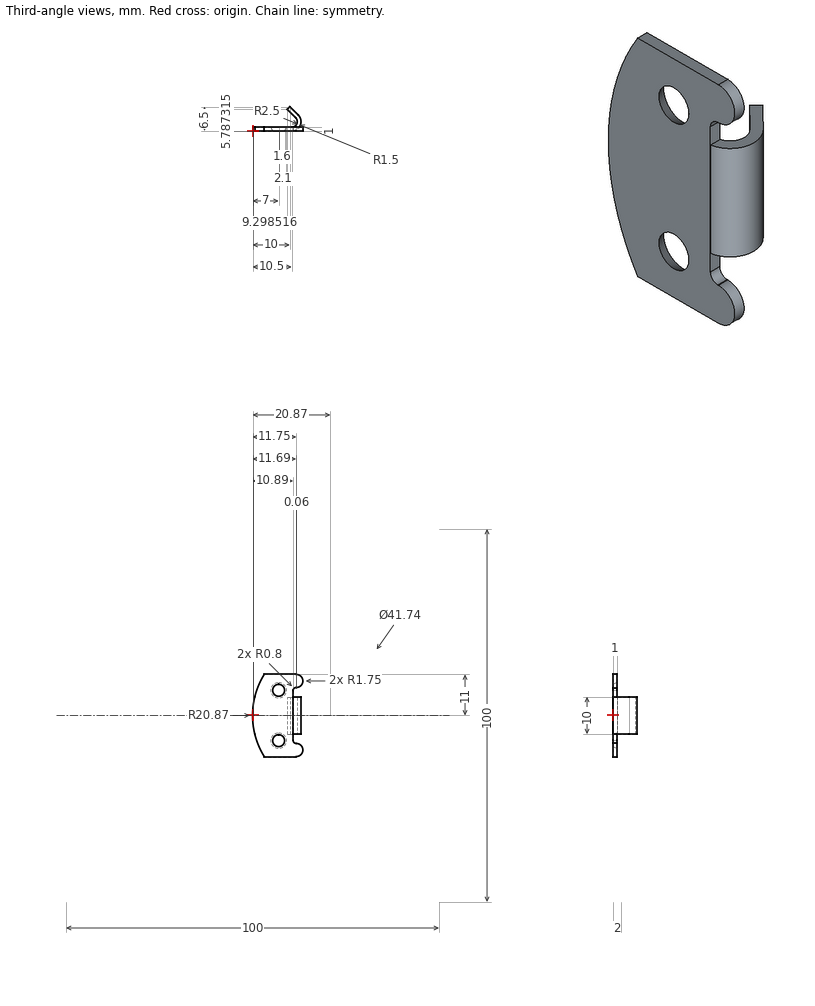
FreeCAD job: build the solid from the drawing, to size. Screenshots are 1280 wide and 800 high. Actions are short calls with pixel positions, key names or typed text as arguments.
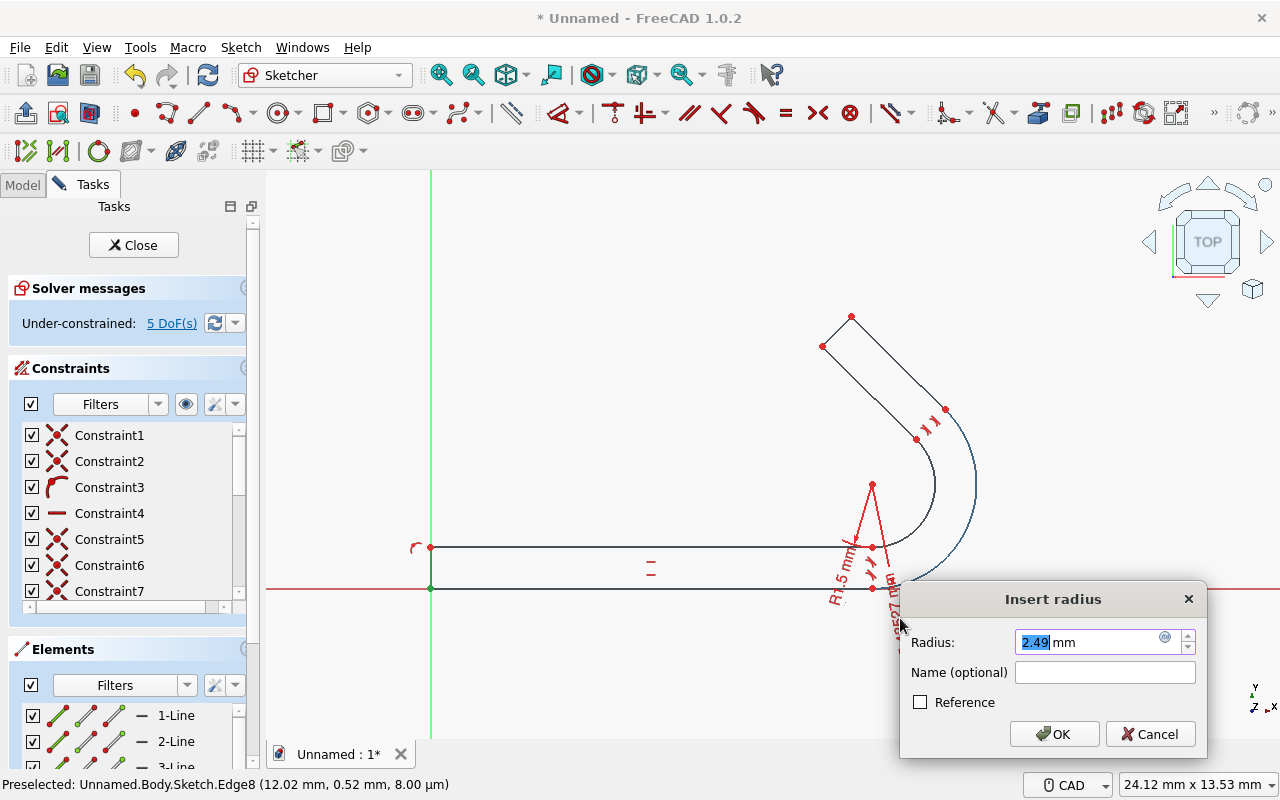
text(2.5)
key(Return)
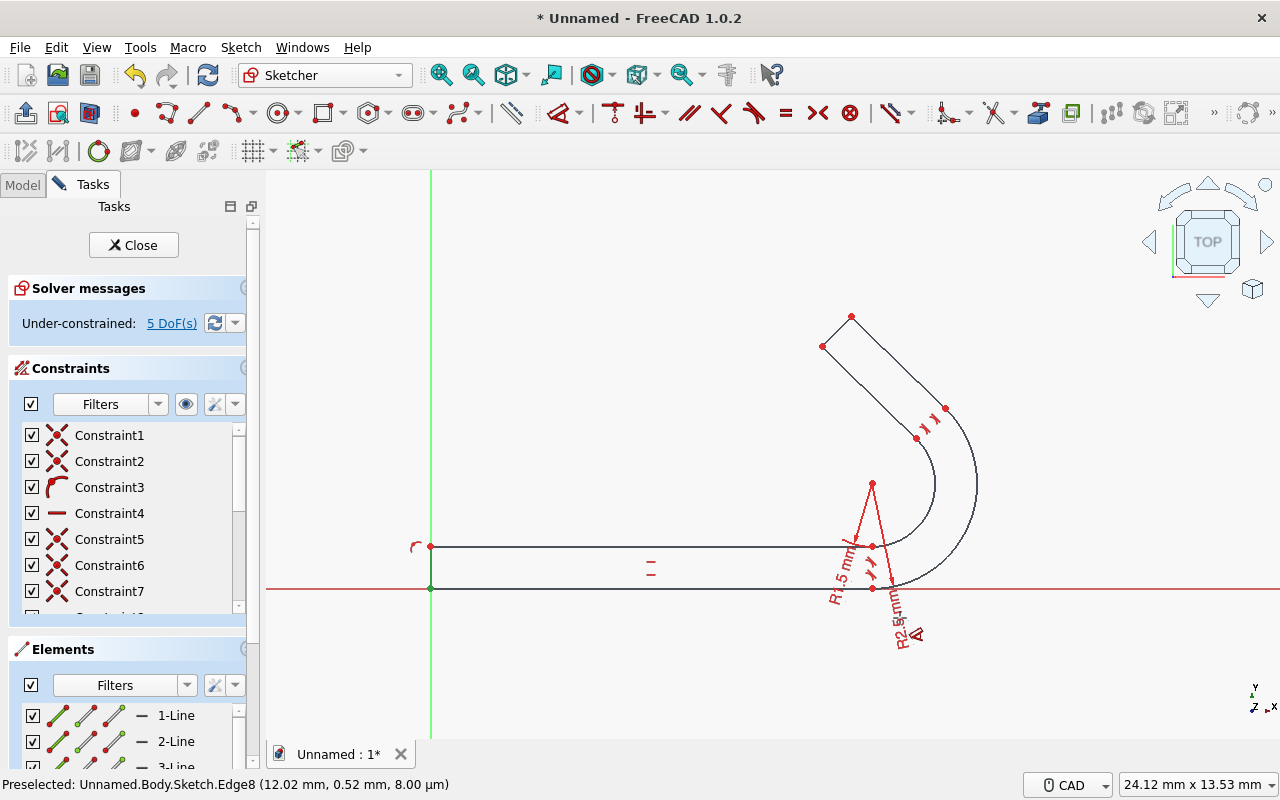
click(851, 317)
click(641, 623)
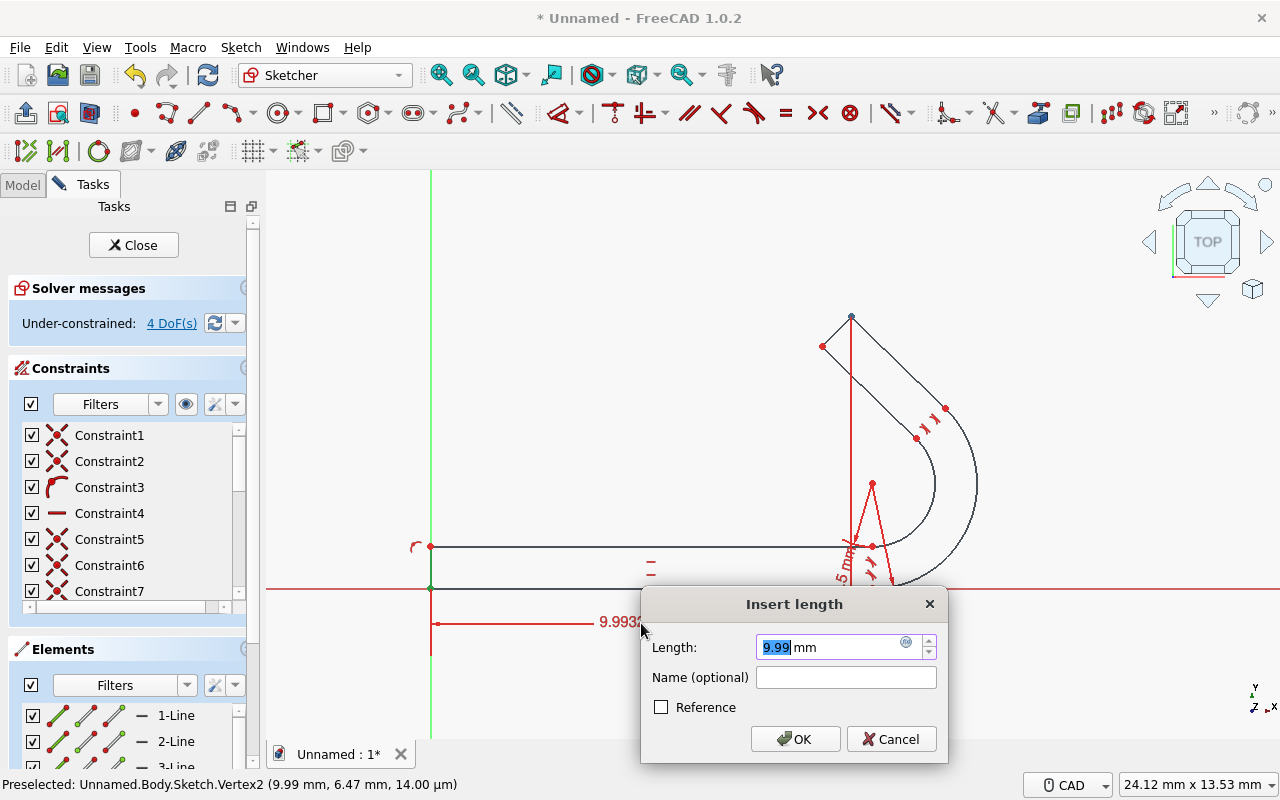
text(10)
key(Return)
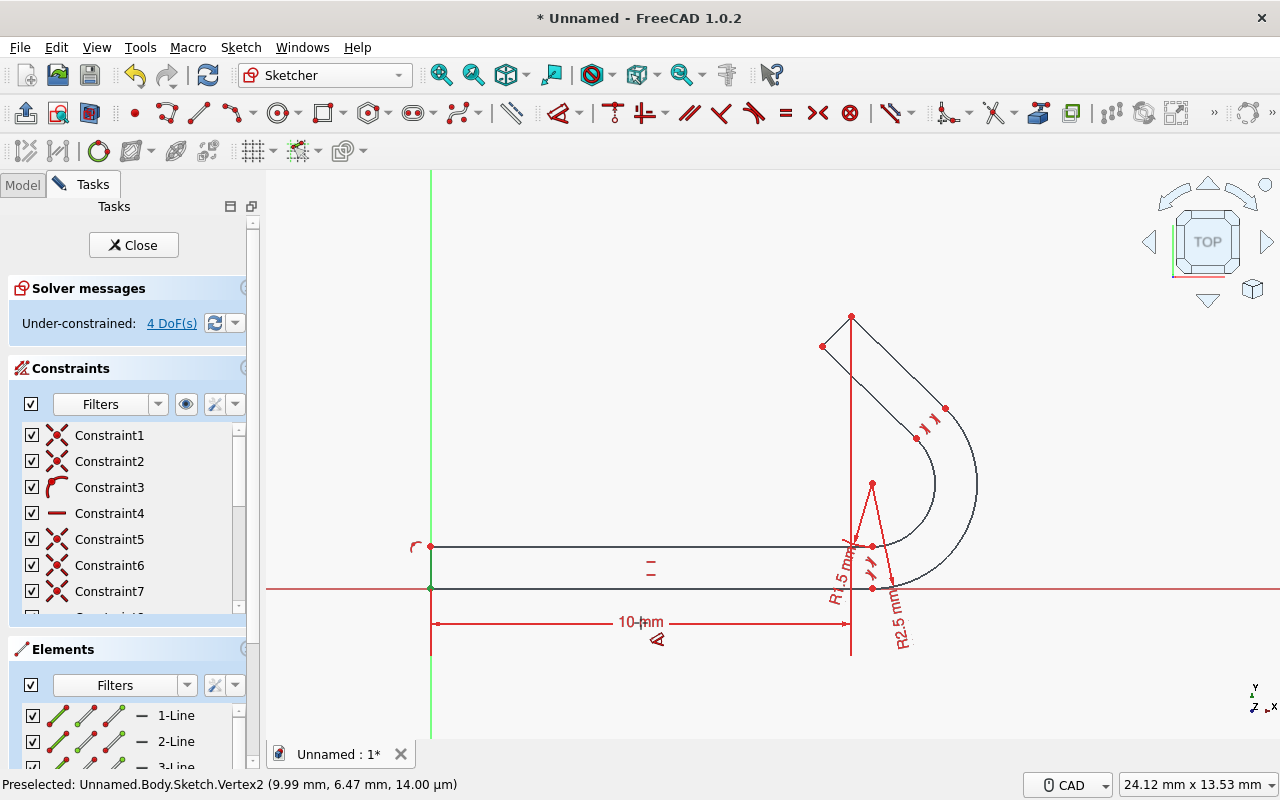
click(740, 547)
click(651, 513)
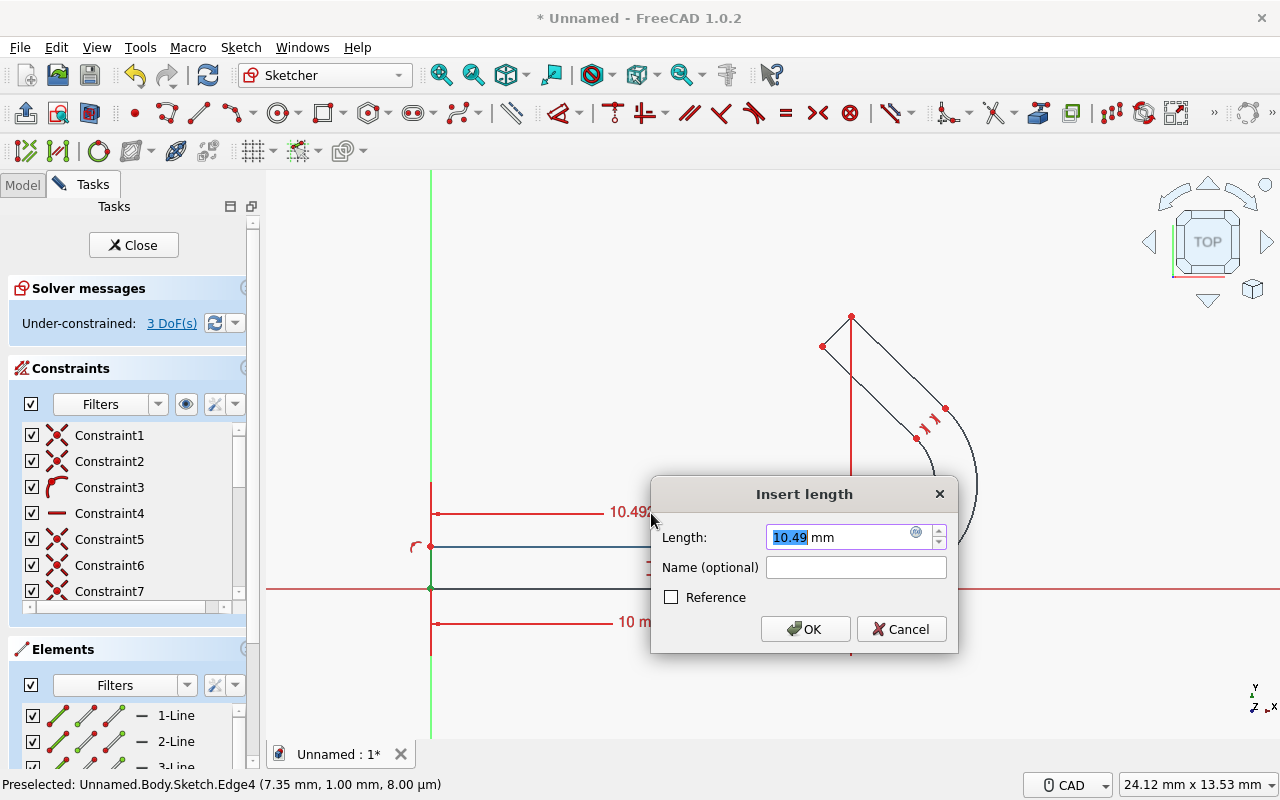
text(10.5)
key(Return)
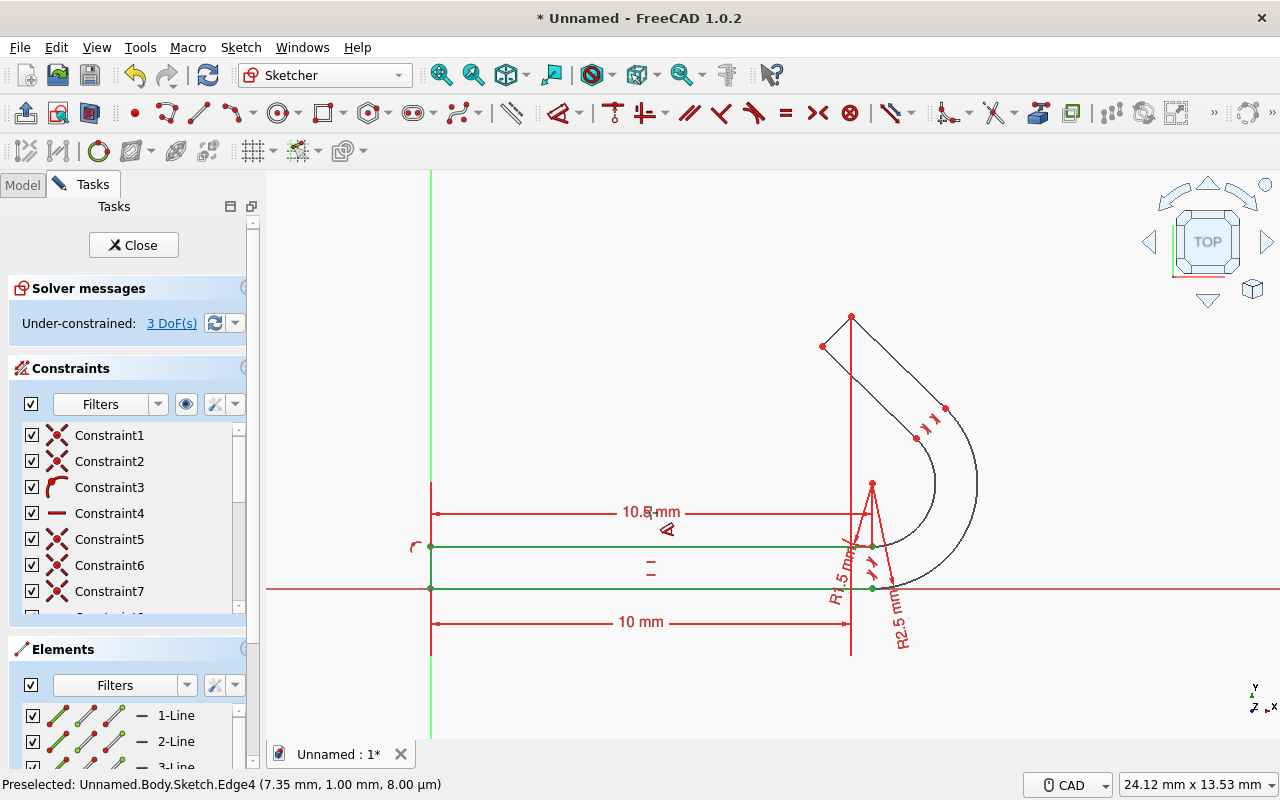
click(851, 317)
click(397, 453)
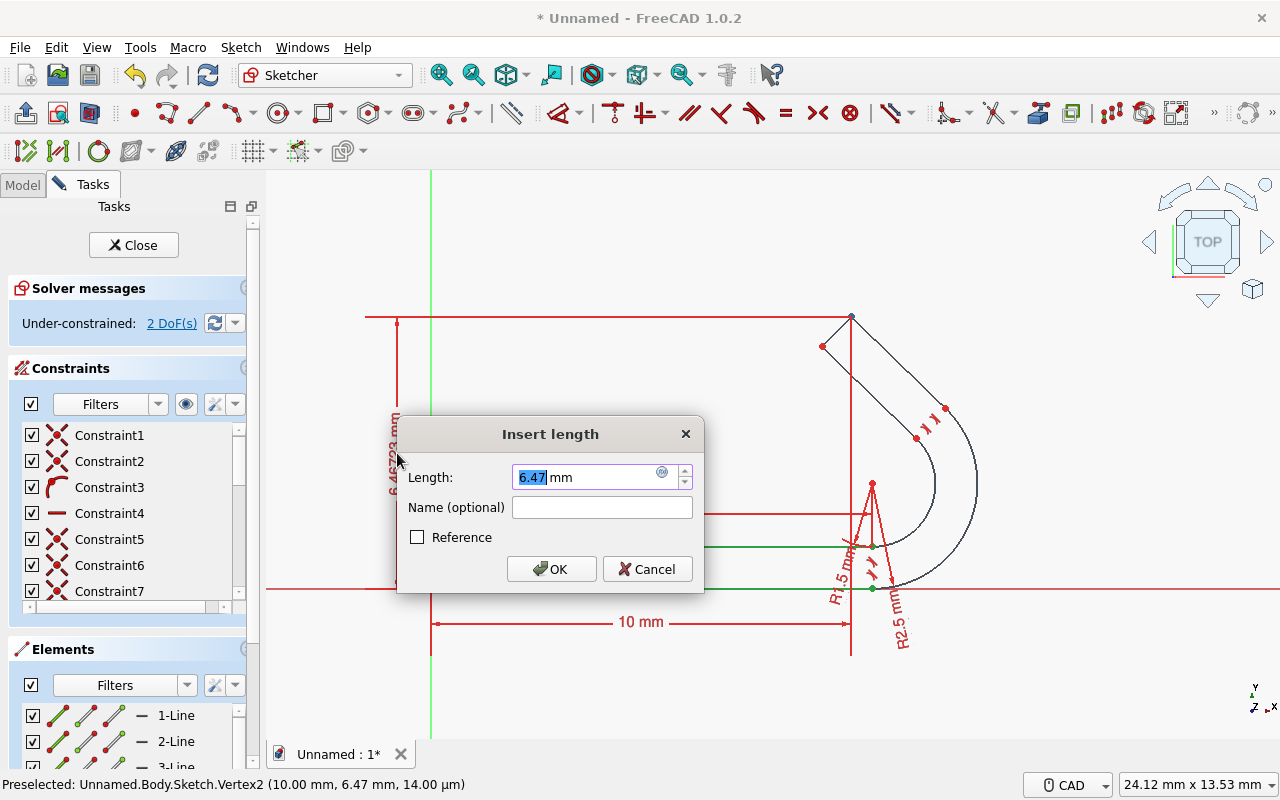
text(6.5)
key(Return)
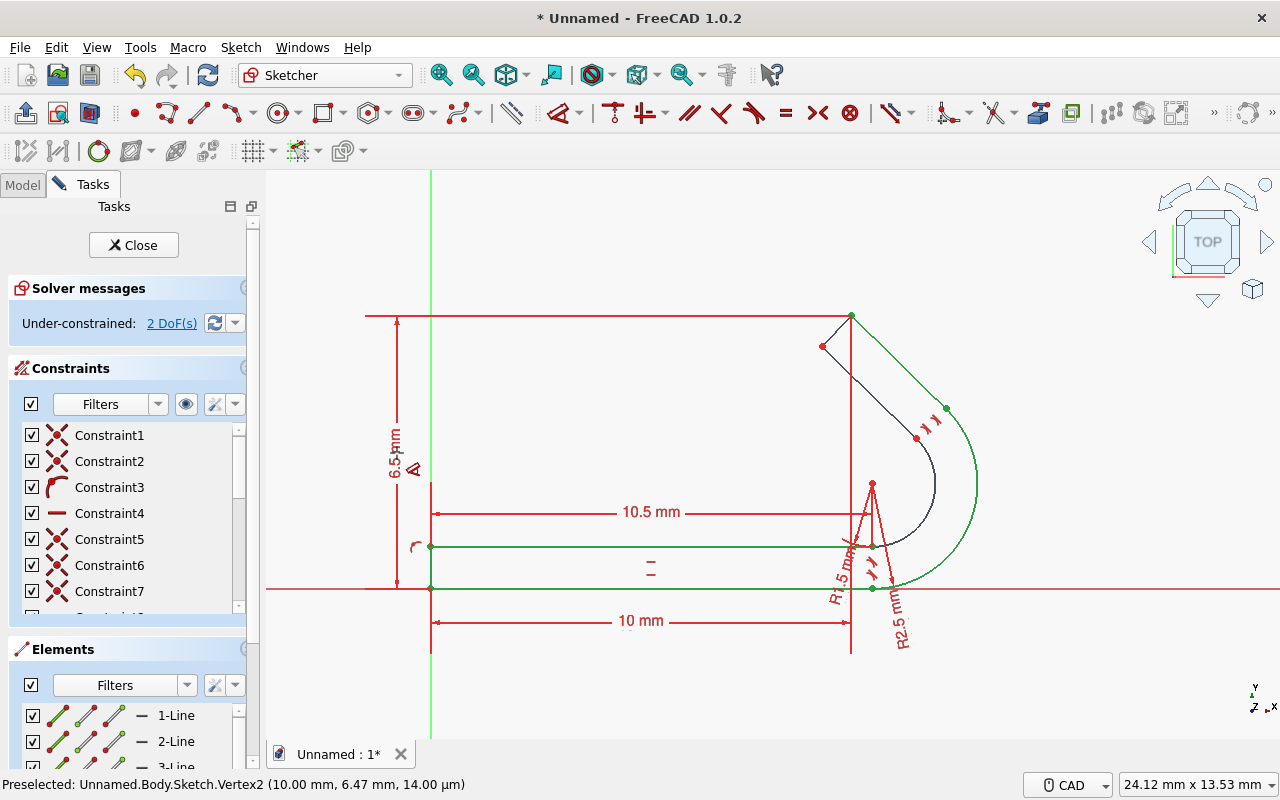
click(822, 347)
click(536, 623)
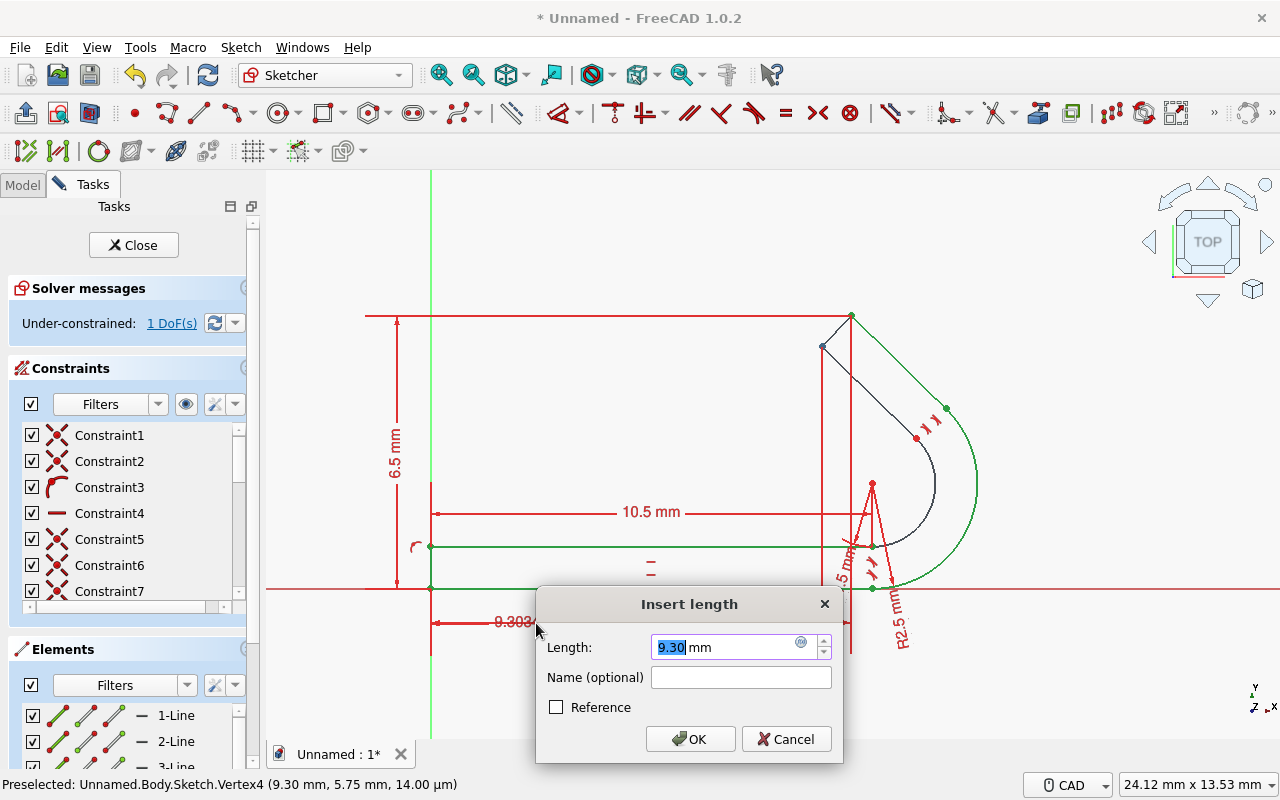
text(9.298516)
key(Return)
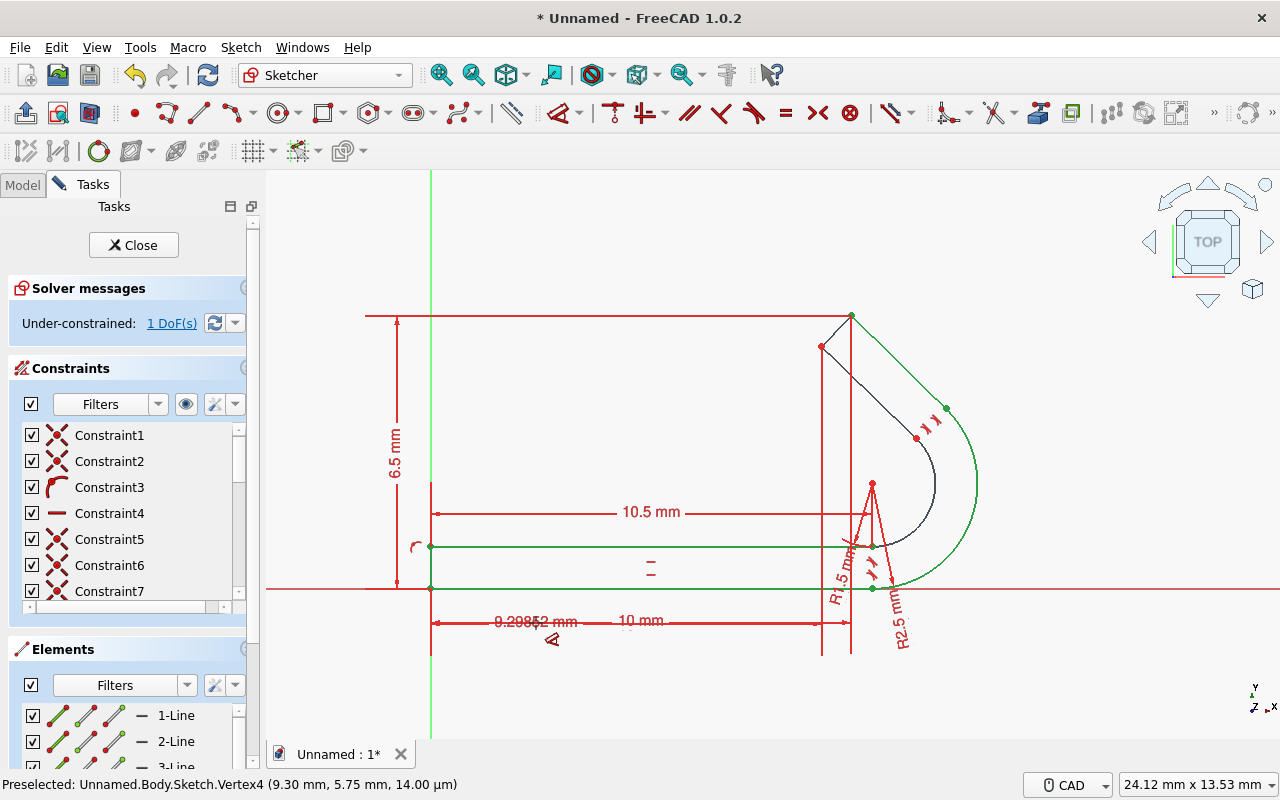
click(822, 347)
click(397, 412)